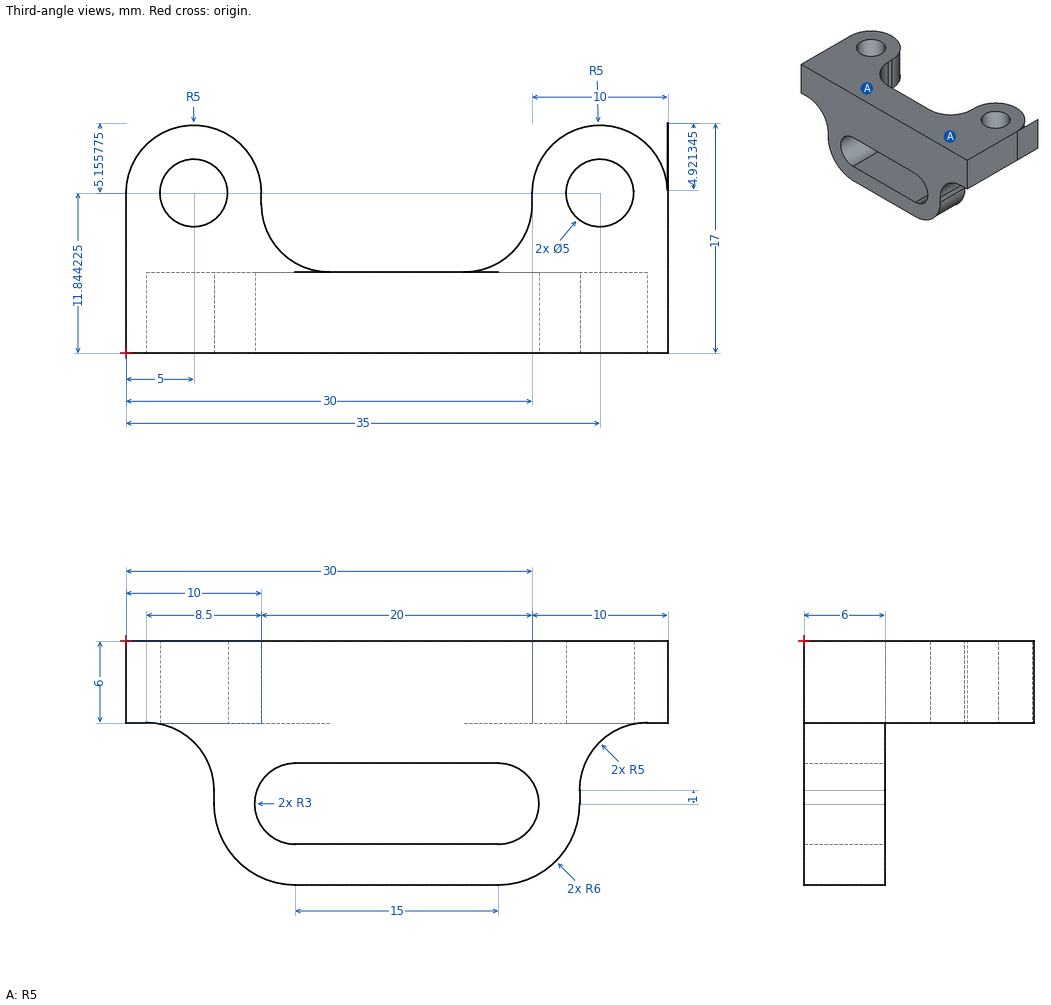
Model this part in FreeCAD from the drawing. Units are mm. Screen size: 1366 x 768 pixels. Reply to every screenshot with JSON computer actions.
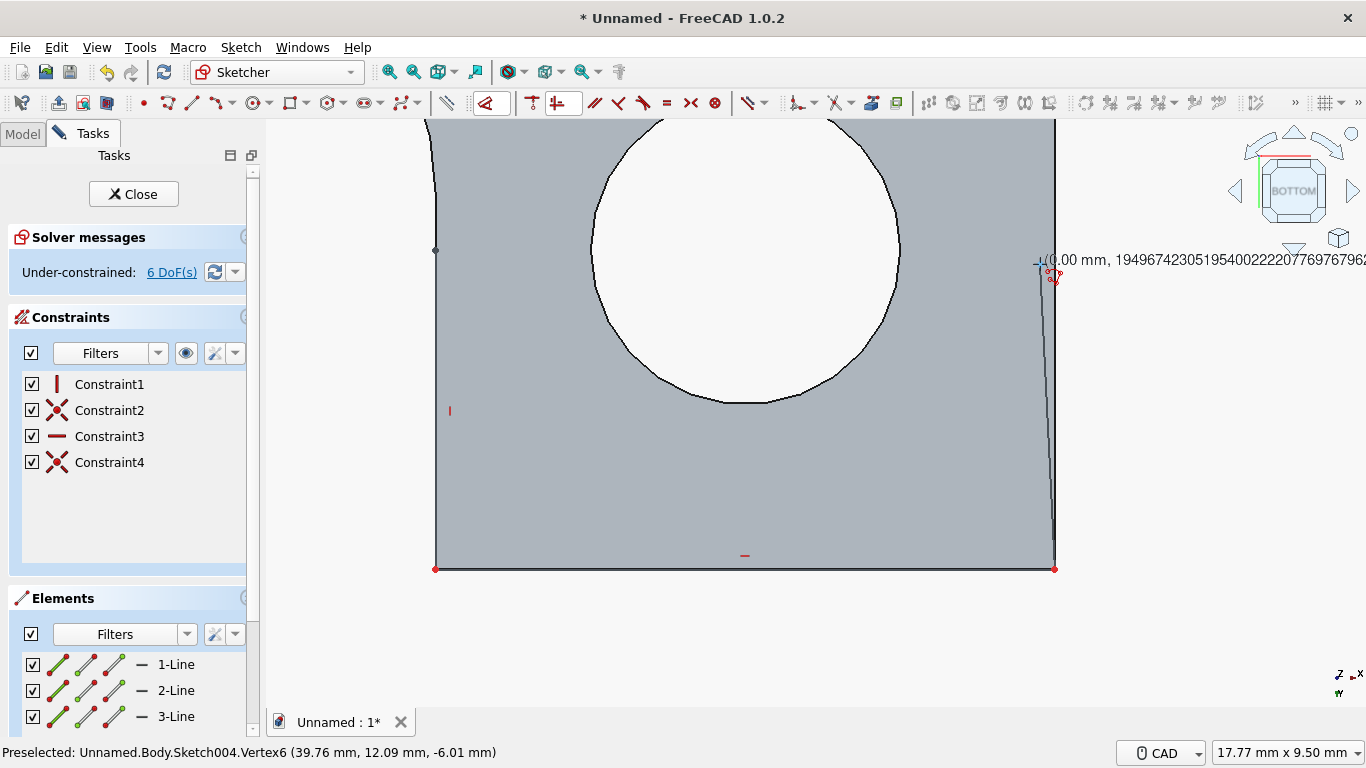
{"action": "key", "text": "g 3 a"}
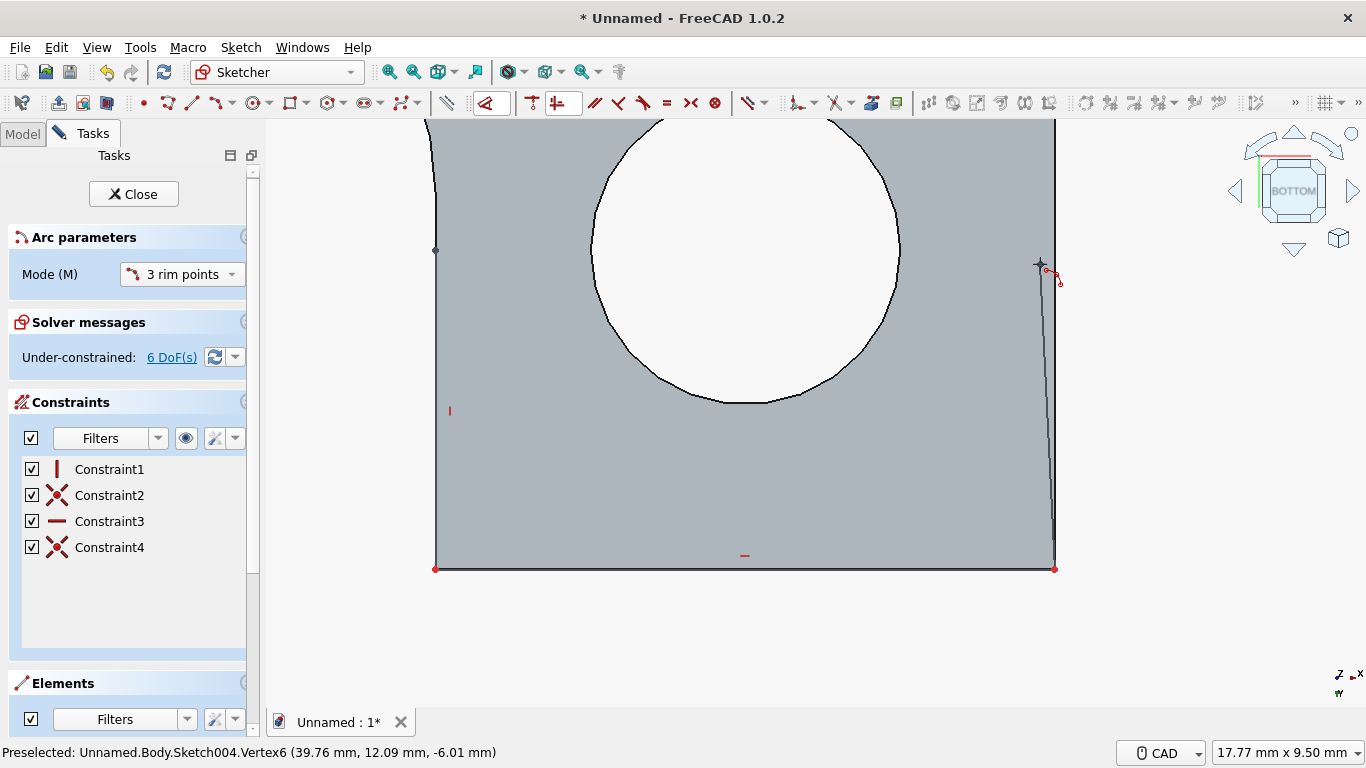
{"action": "left_click", "coordinate": [1040, 265]}
{"action": "left_click", "coordinate": [436, 251]}
{"action": "left_click", "coordinate": [644, 542]}
{"action": "key", "text": "Escape"}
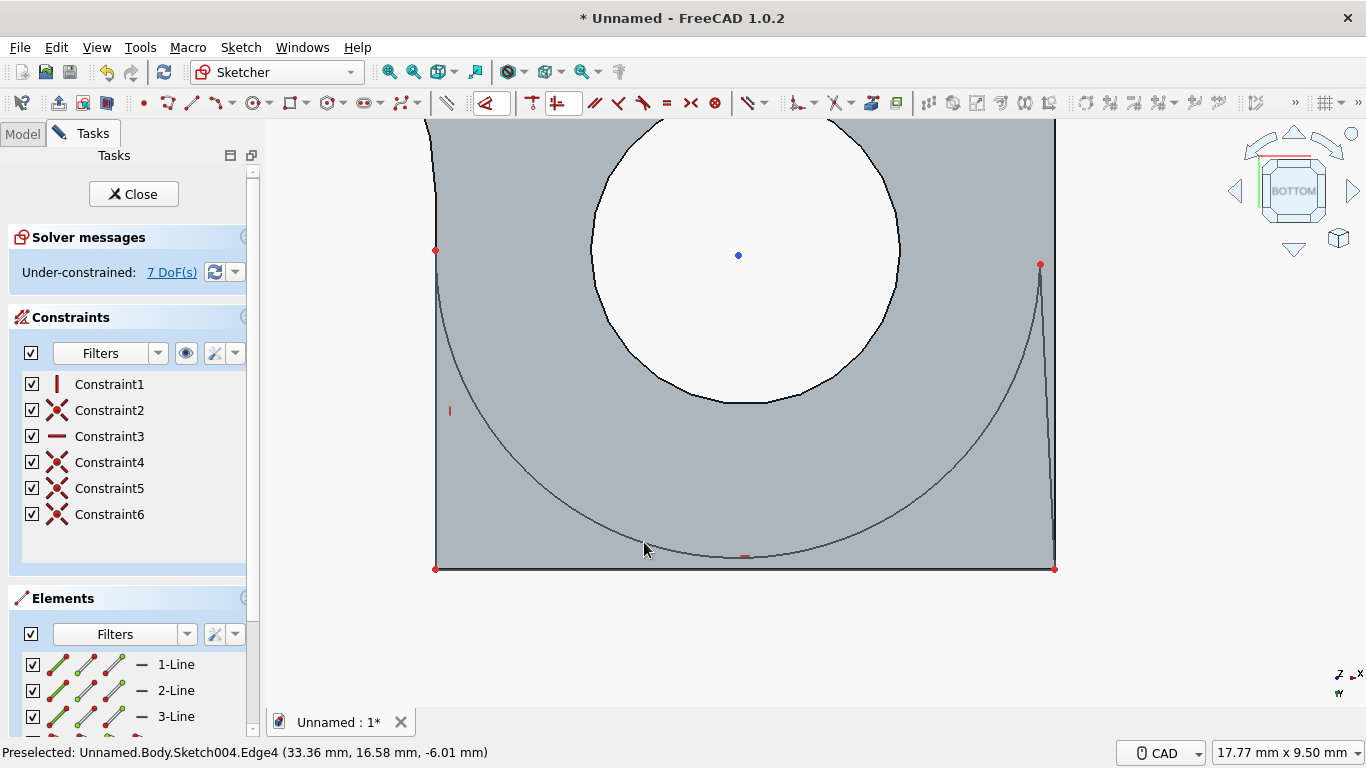
{"action": "left_click", "coordinate": [436, 347]}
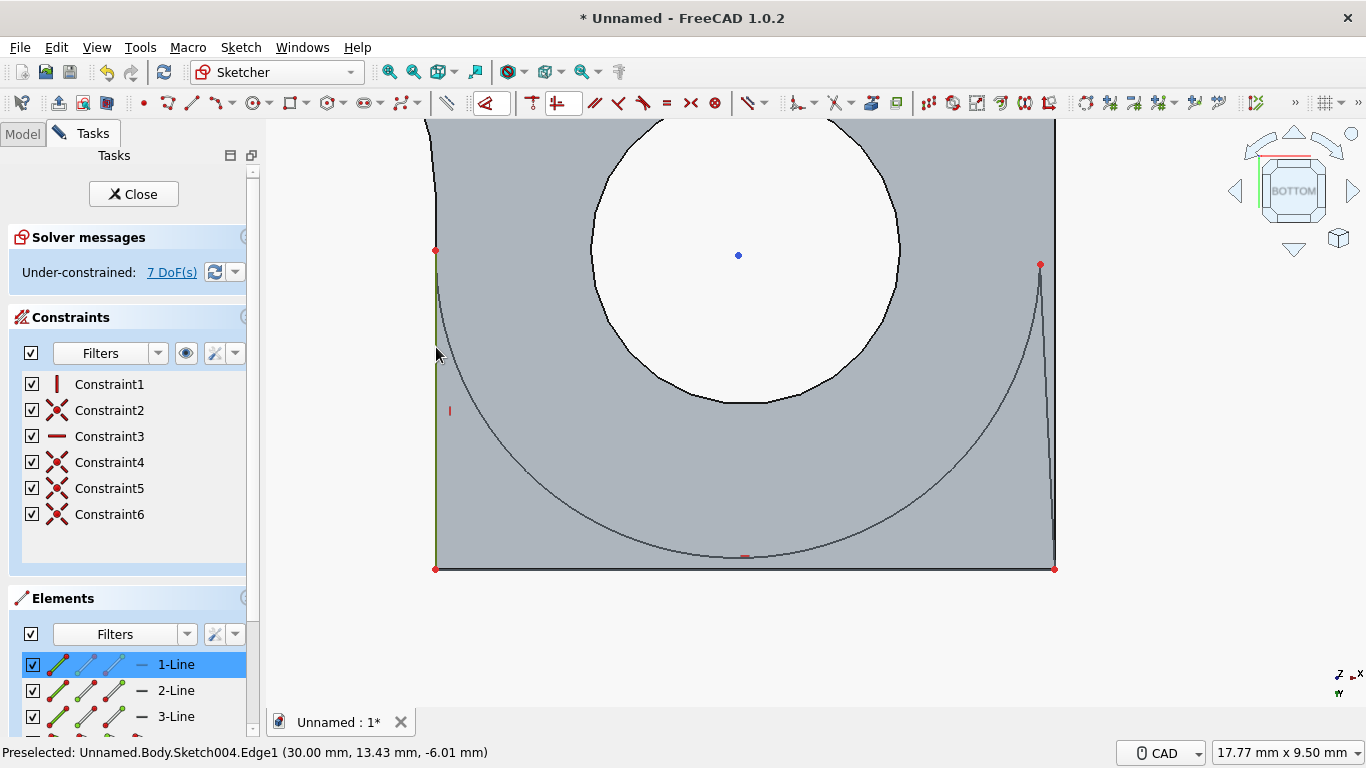
{"action": "left_click", "coordinate": [556, 497]}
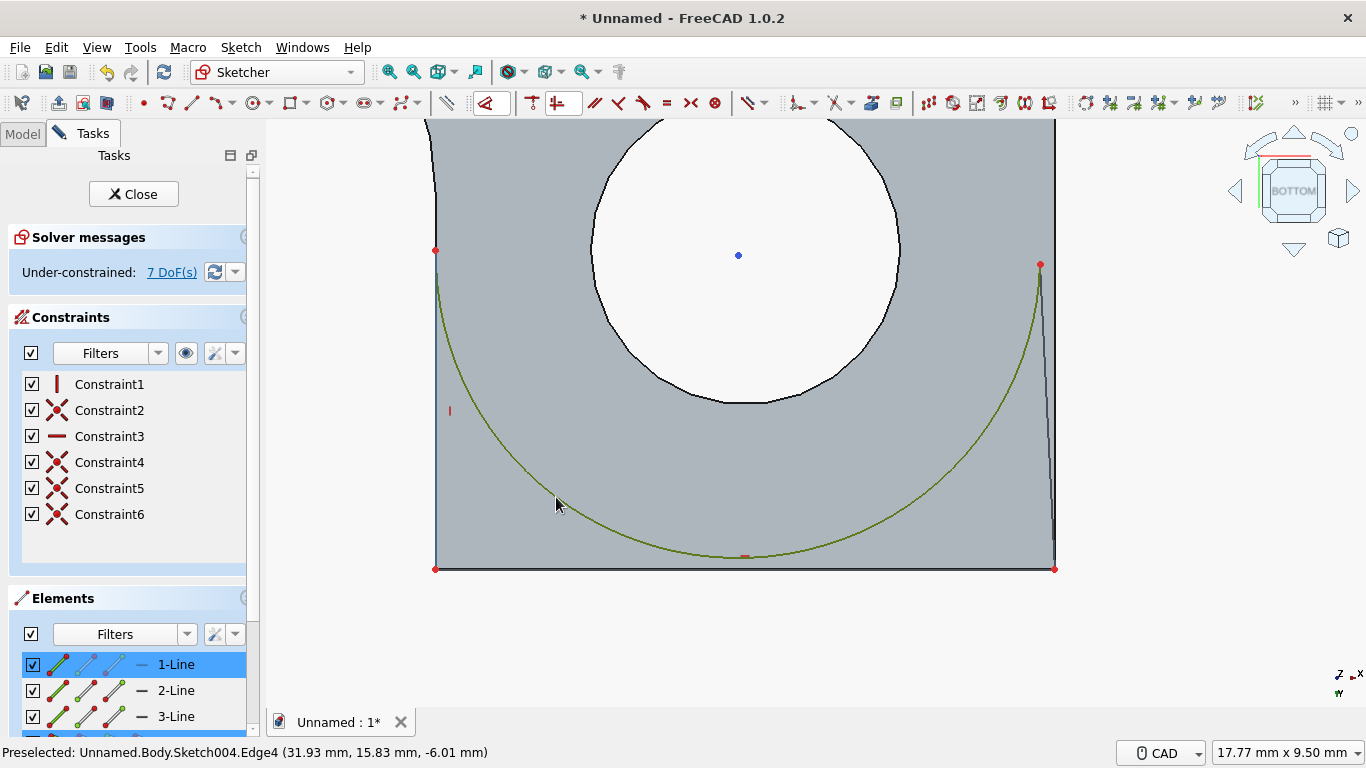
{"action": "key", "text": "t"}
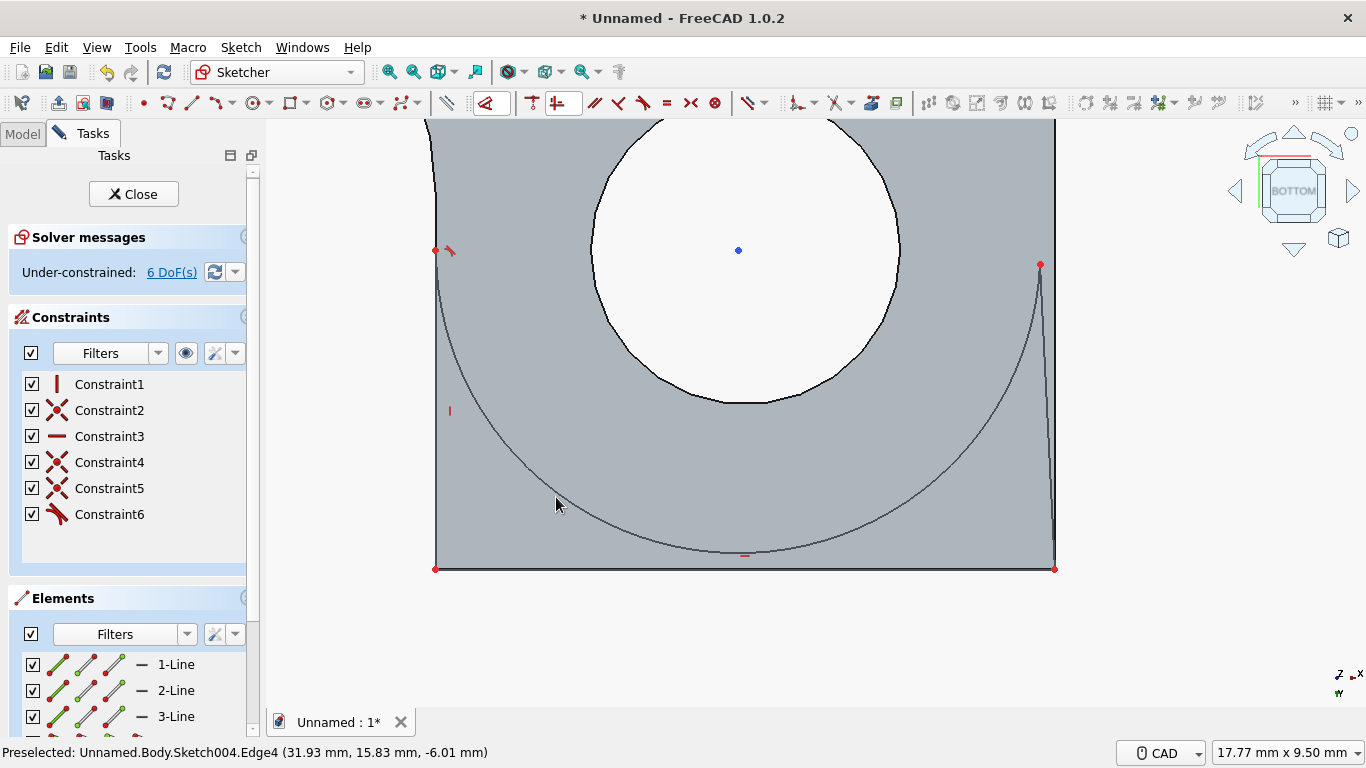
{"action": "left_click", "coordinate": [557, 493]}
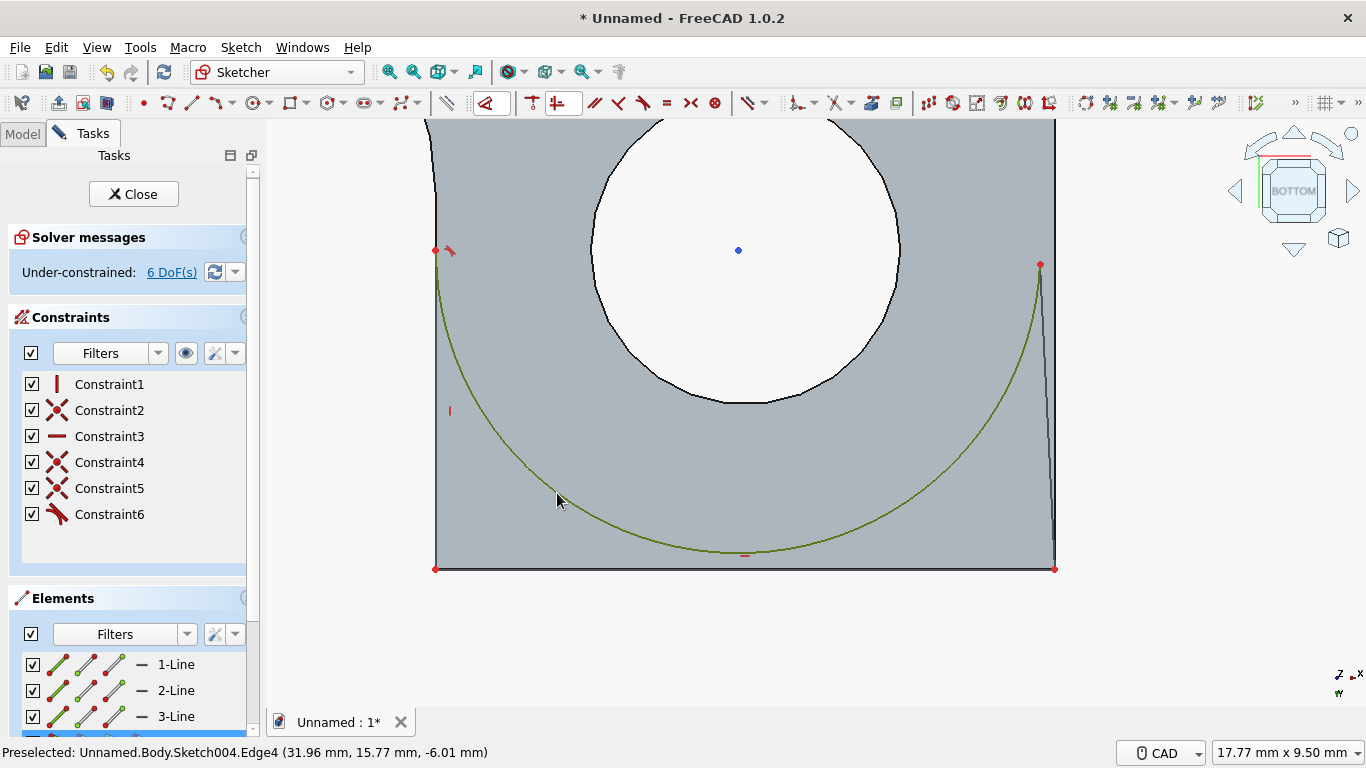
{"action": "key", "text": "k r"}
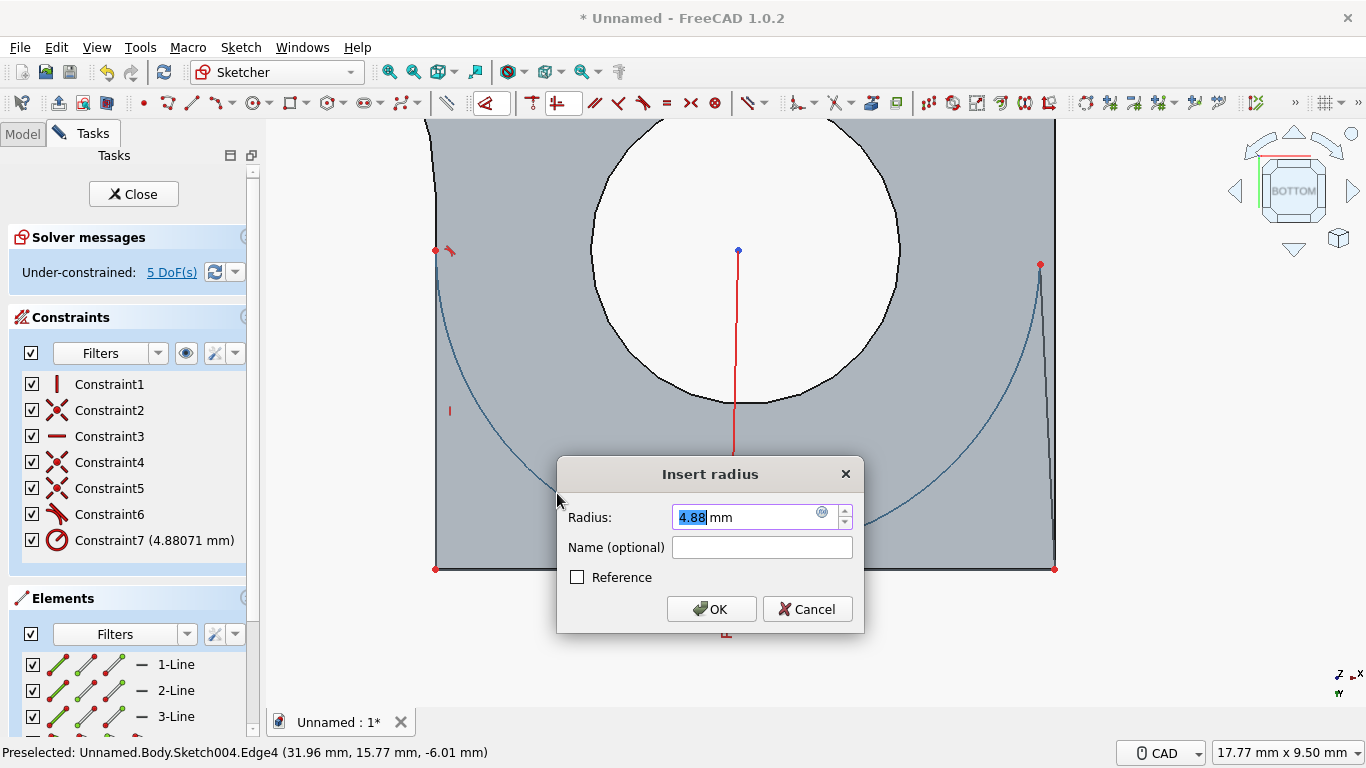
{"action": "type", "text": "5"}
{"action": "key", "text": "Return"}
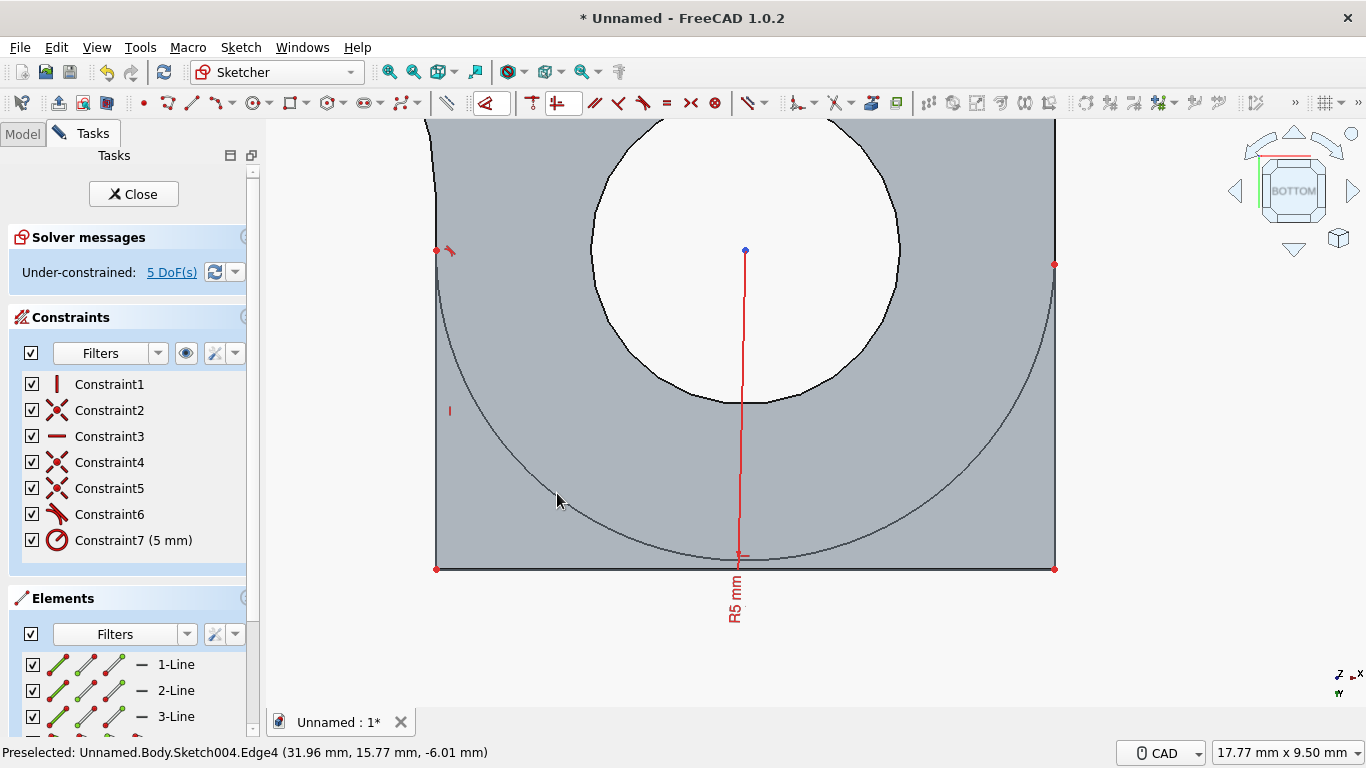
{"action": "left_click", "coordinate": [622, 570]}